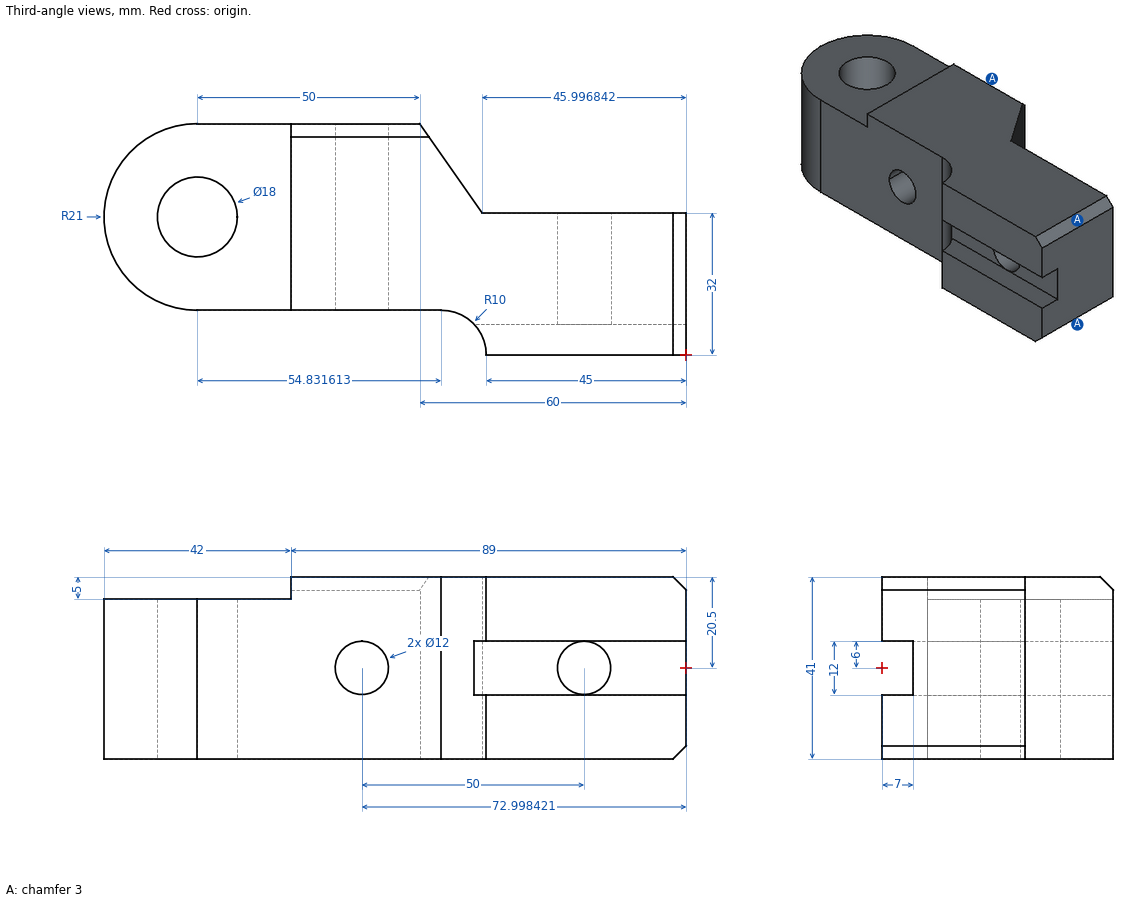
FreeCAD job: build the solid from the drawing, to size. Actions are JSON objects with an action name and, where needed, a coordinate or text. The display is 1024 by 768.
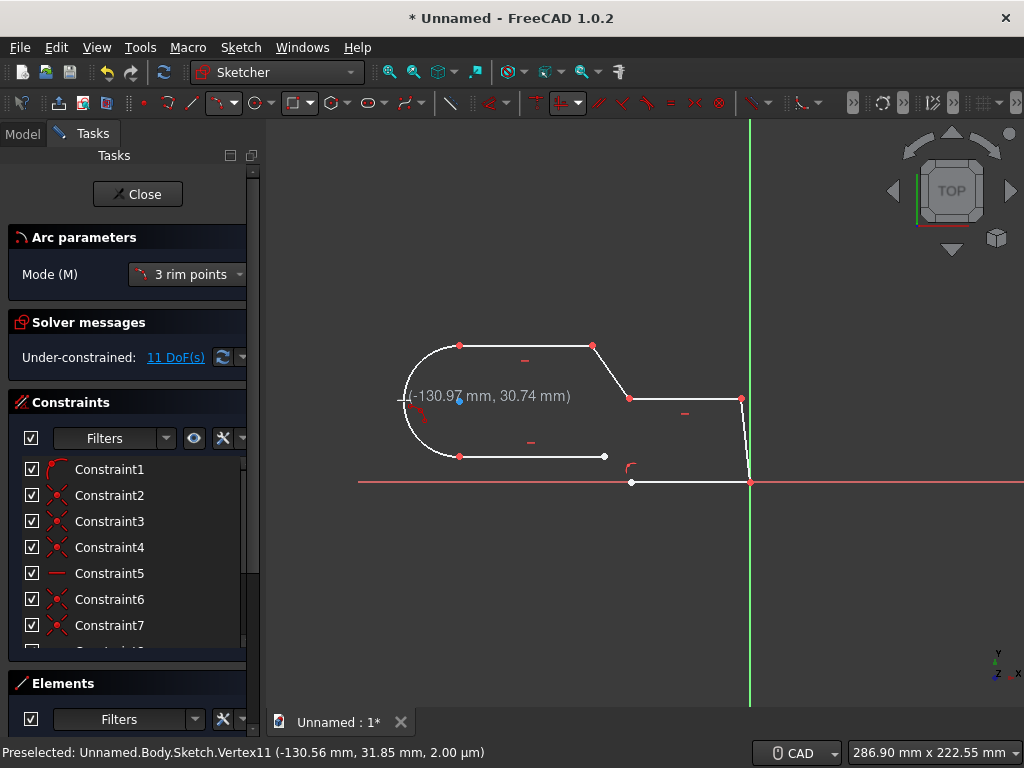
{"action": "left_click", "coordinate": [604, 457]}
{"action": "left_click", "coordinate": [631, 482]}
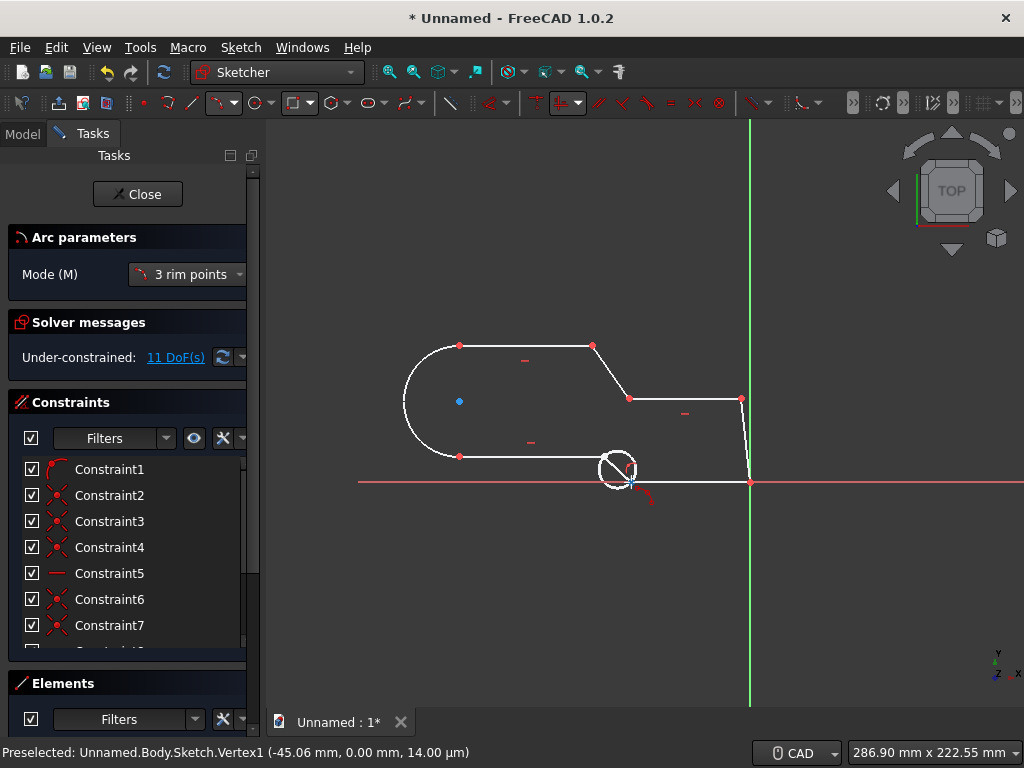
{"action": "scroll", "coordinate": [623, 463], "scroll_direction": "up", "scroll_amount": 4}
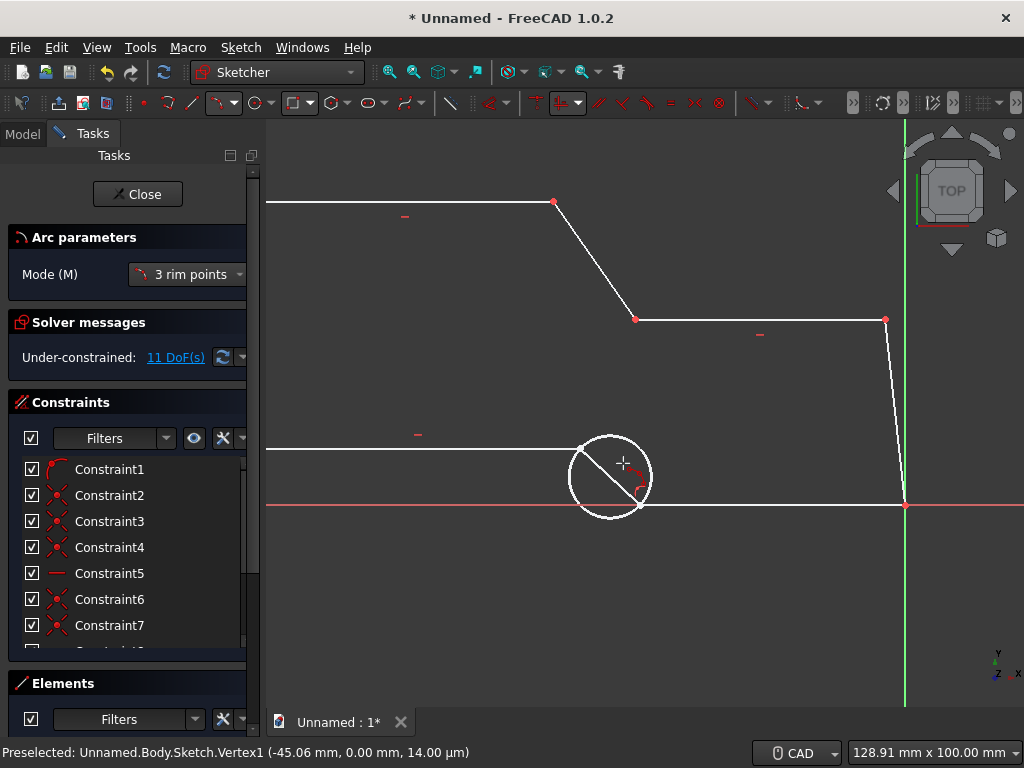
{"action": "left_click", "coordinate": [623, 463]}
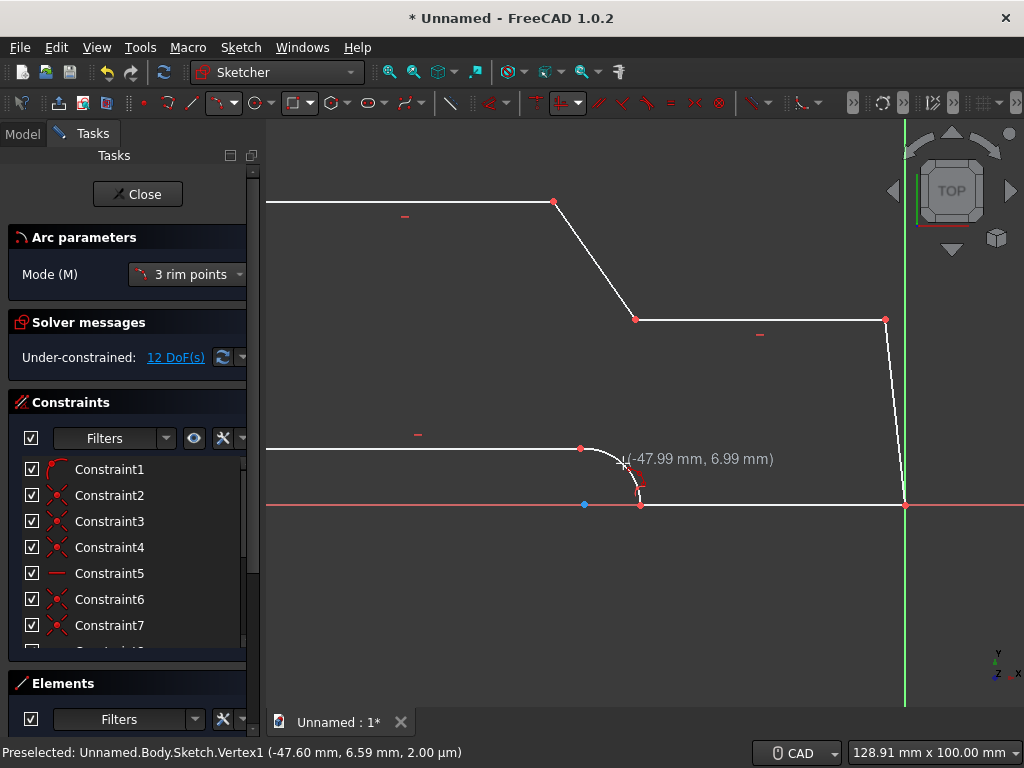
{"action": "left_click", "coordinate": [256, 104]}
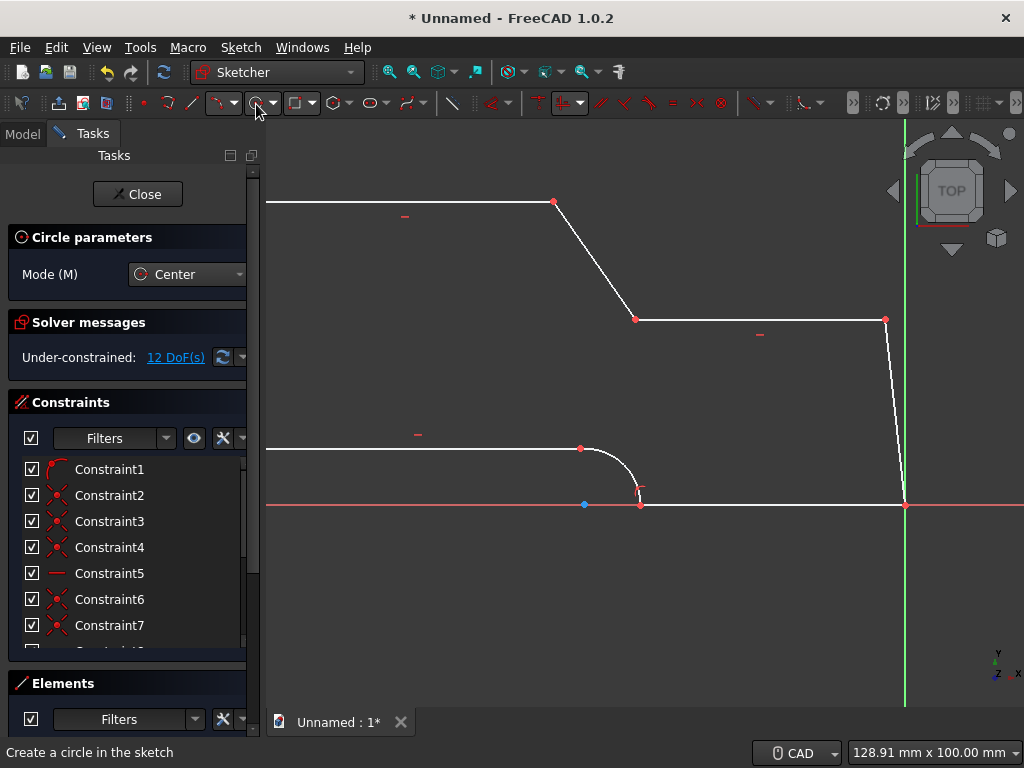
{"action": "scroll", "coordinate": [645, 487], "scroll_direction": "down", "scroll_amount": 3}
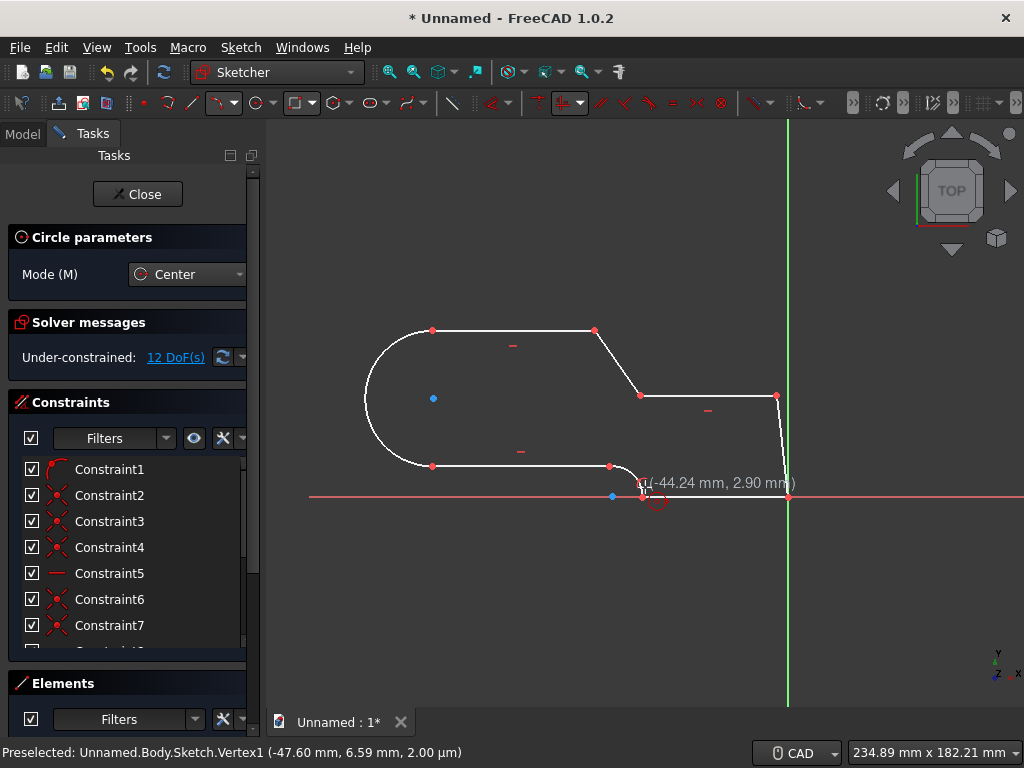
{"action": "left_click", "coordinate": [433, 397]}
{"action": "left_click", "coordinate": [454, 377]}
{"action": "key", "text": "Escape"}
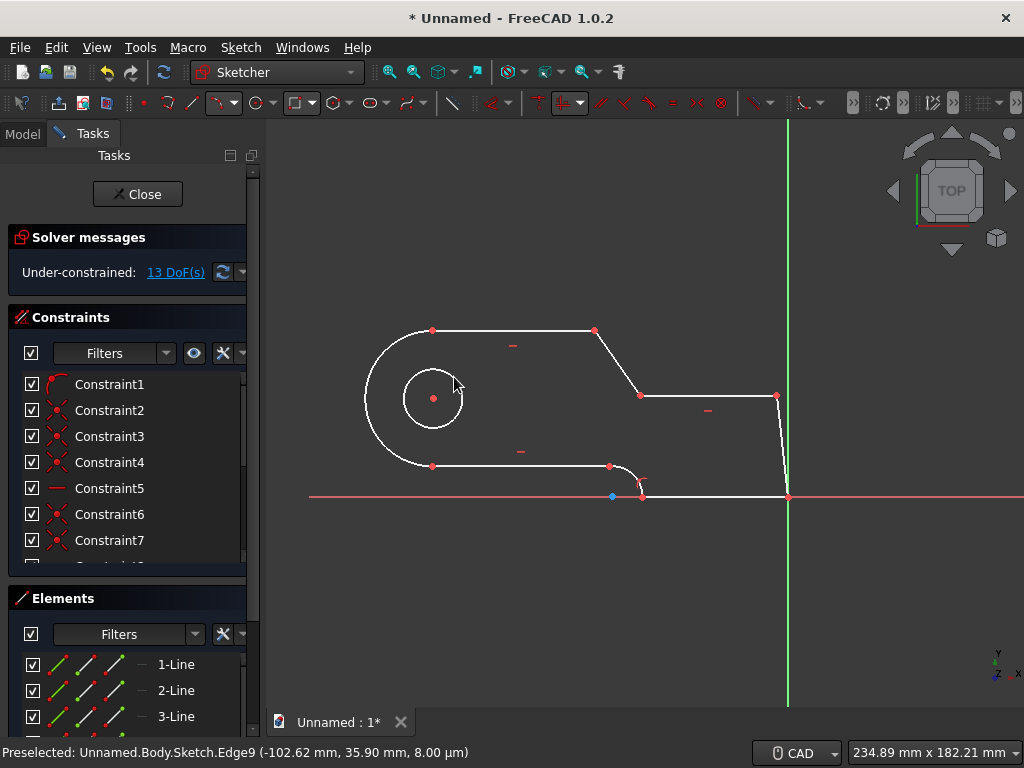
{"action": "left_click", "coordinate": [546, 331]}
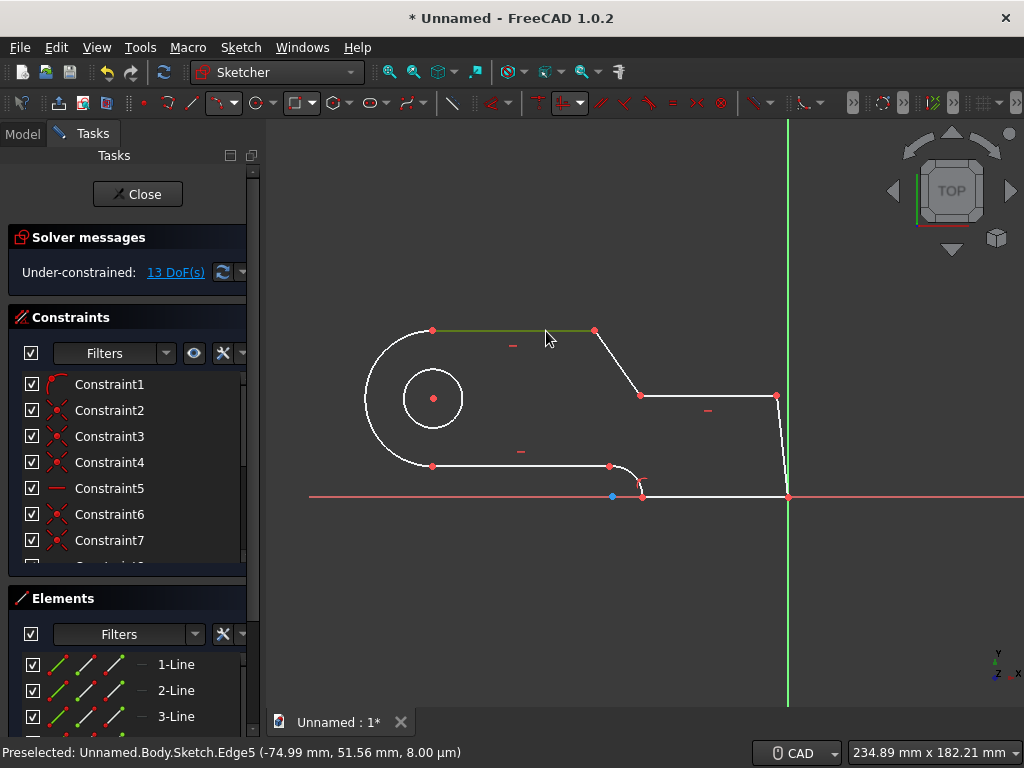
{"action": "left_click", "coordinate": [378, 359]}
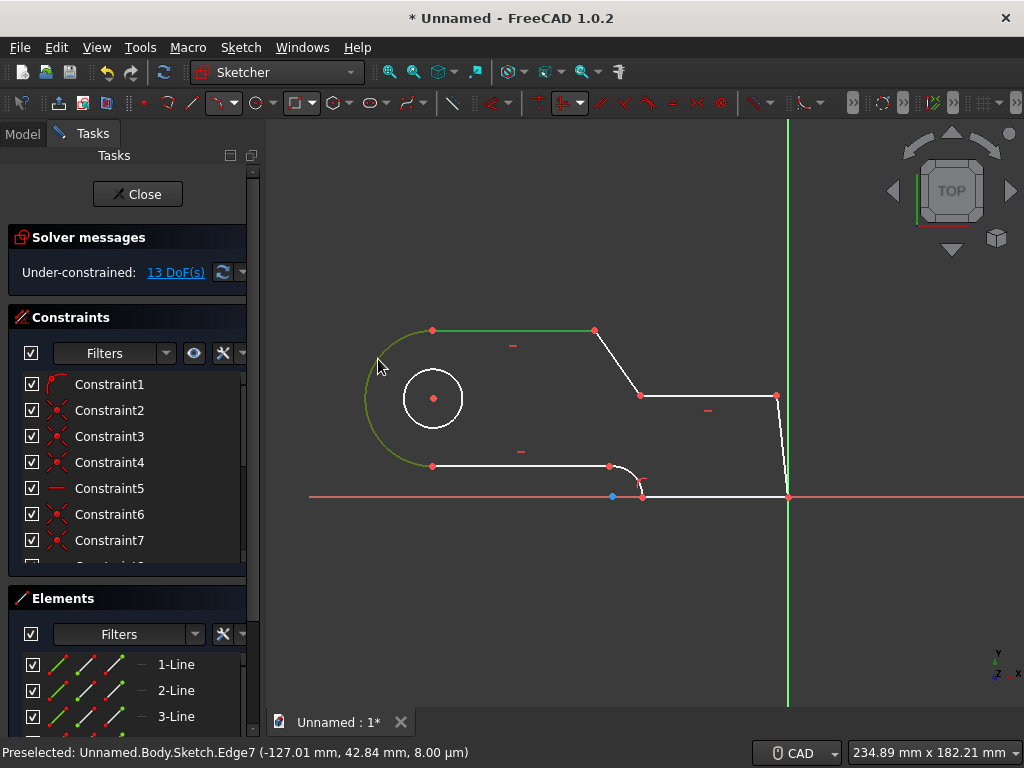
{"action": "left_click", "coordinate": [650, 104]}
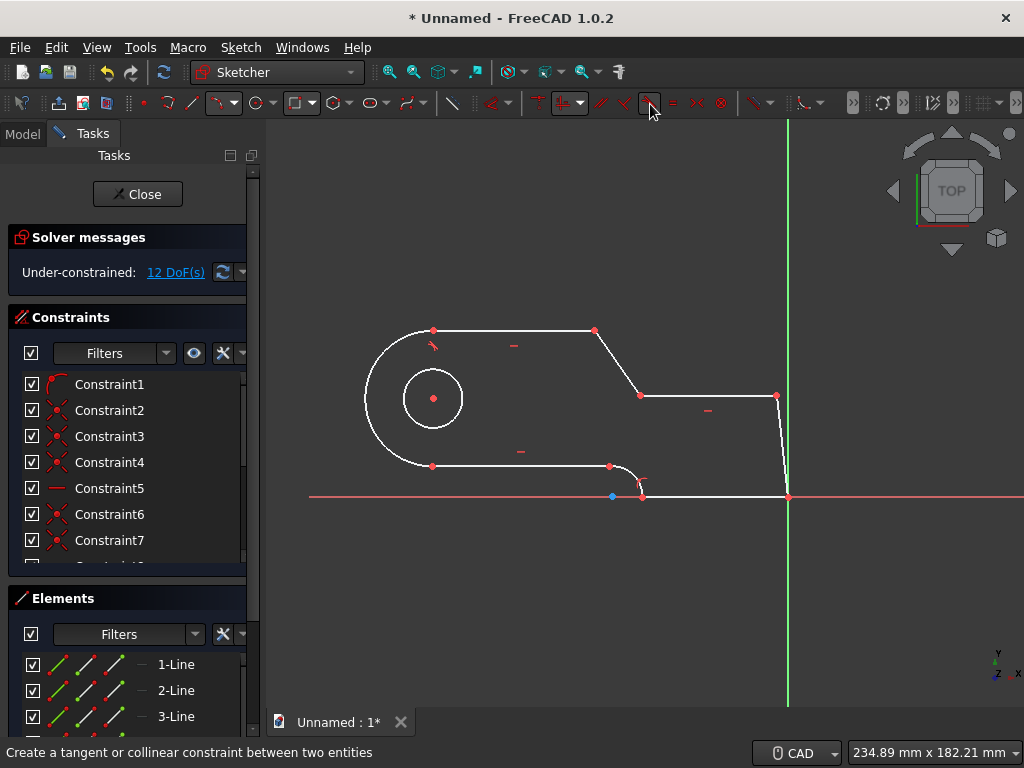
{"action": "left_click", "coordinate": [486, 466]}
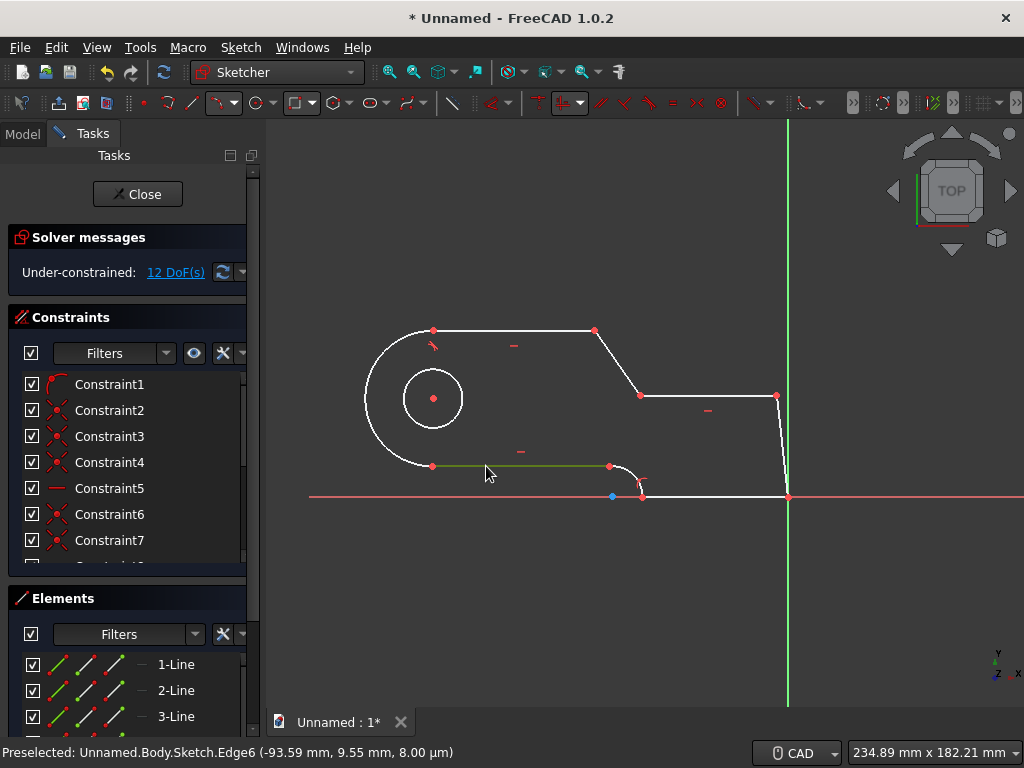
{"action": "left_click", "coordinate": [378, 359]}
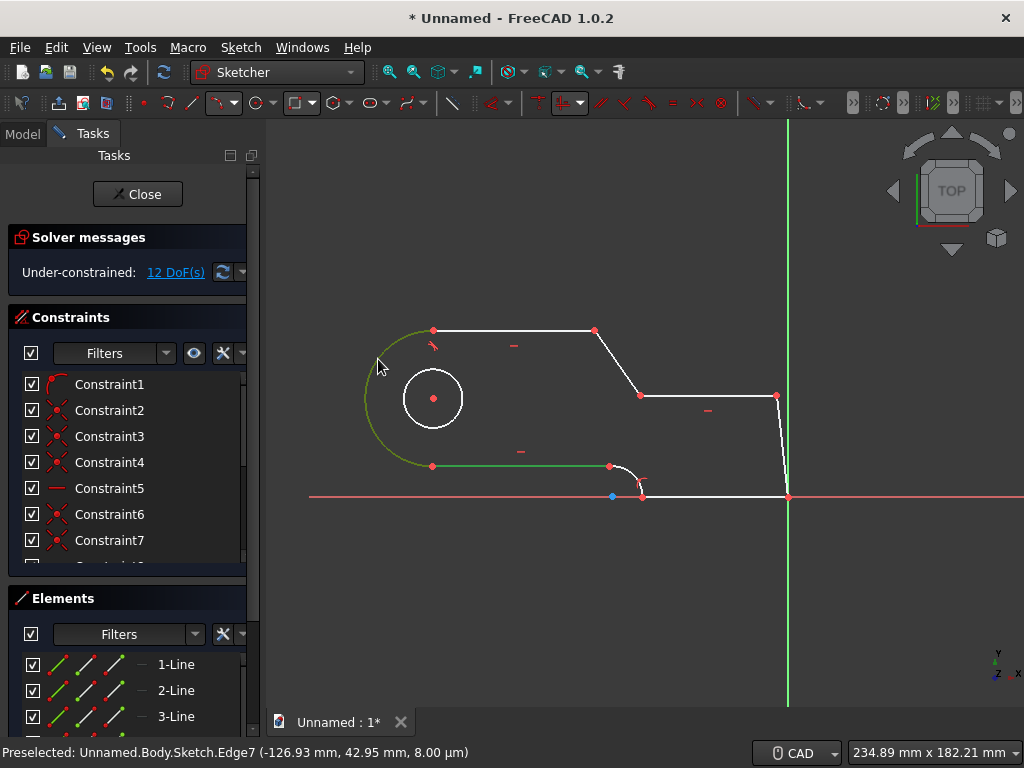
{"action": "left_click", "coordinate": [650, 104]}